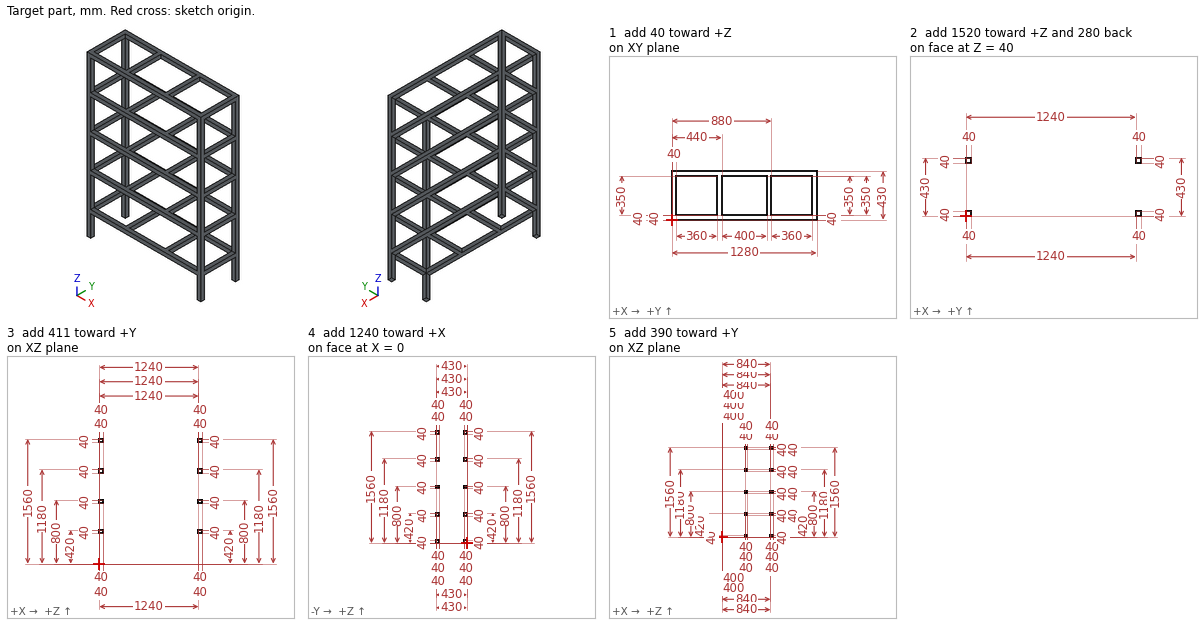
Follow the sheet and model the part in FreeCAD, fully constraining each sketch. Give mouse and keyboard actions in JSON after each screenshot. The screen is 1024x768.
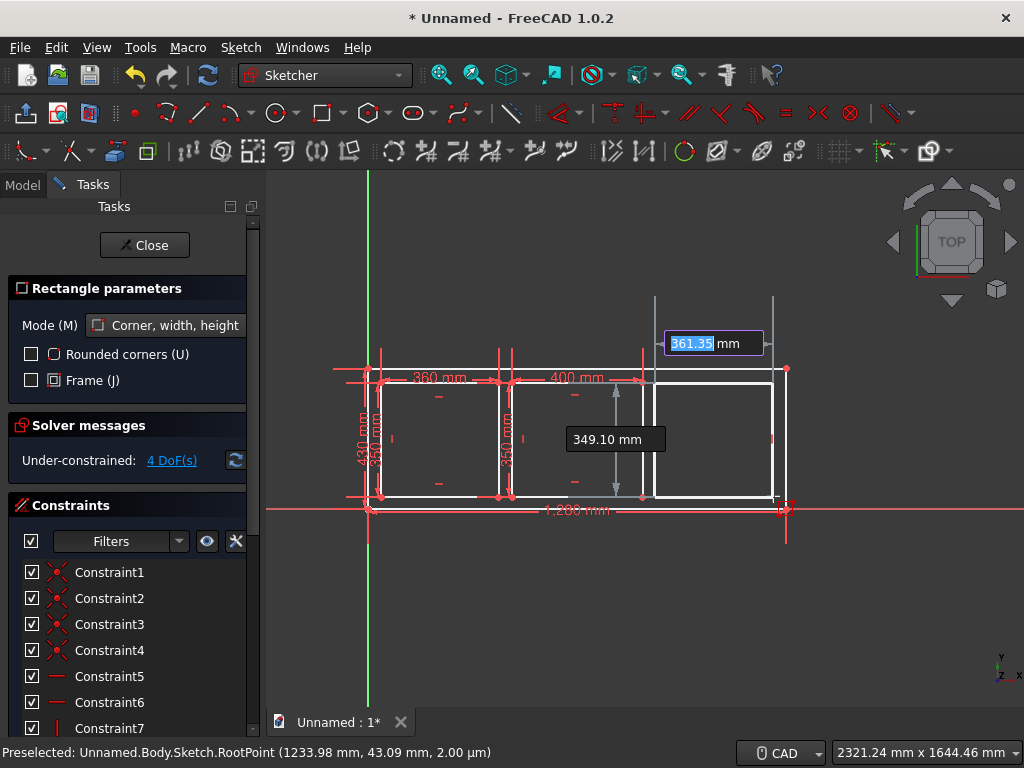
{"action": "type", "text": "360"}
{"action": "key", "text": "Tab"}
{"action": "type", "text": "350"}
{"action": "key", "text": "Return"}
{"action": "key", "text": "Escape"}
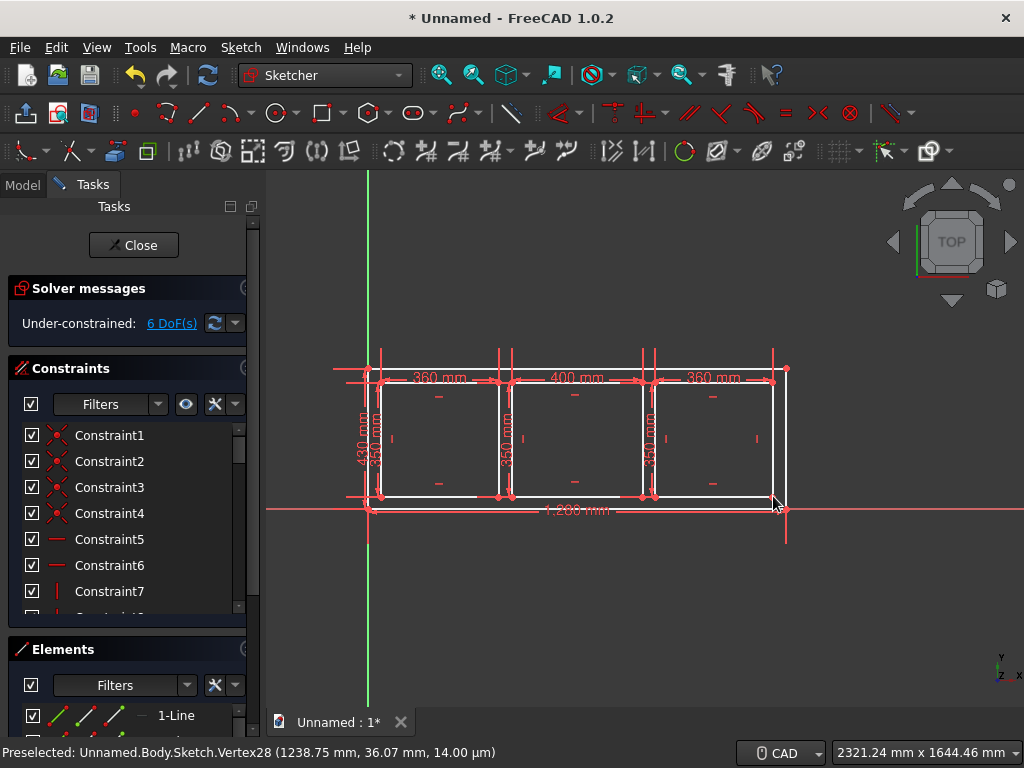
{"action": "left_click", "coordinate": [558, 114]}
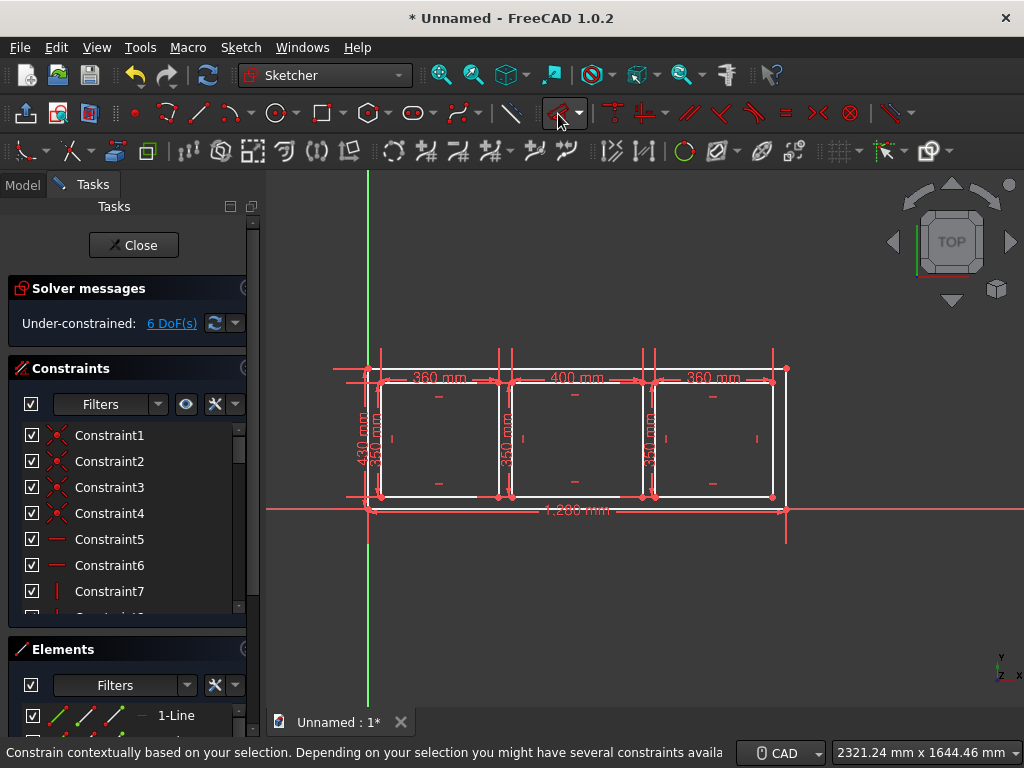
{"action": "scroll", "coordinate": [381, 383], "scroll_direction": "up", "scroll_amount": 6}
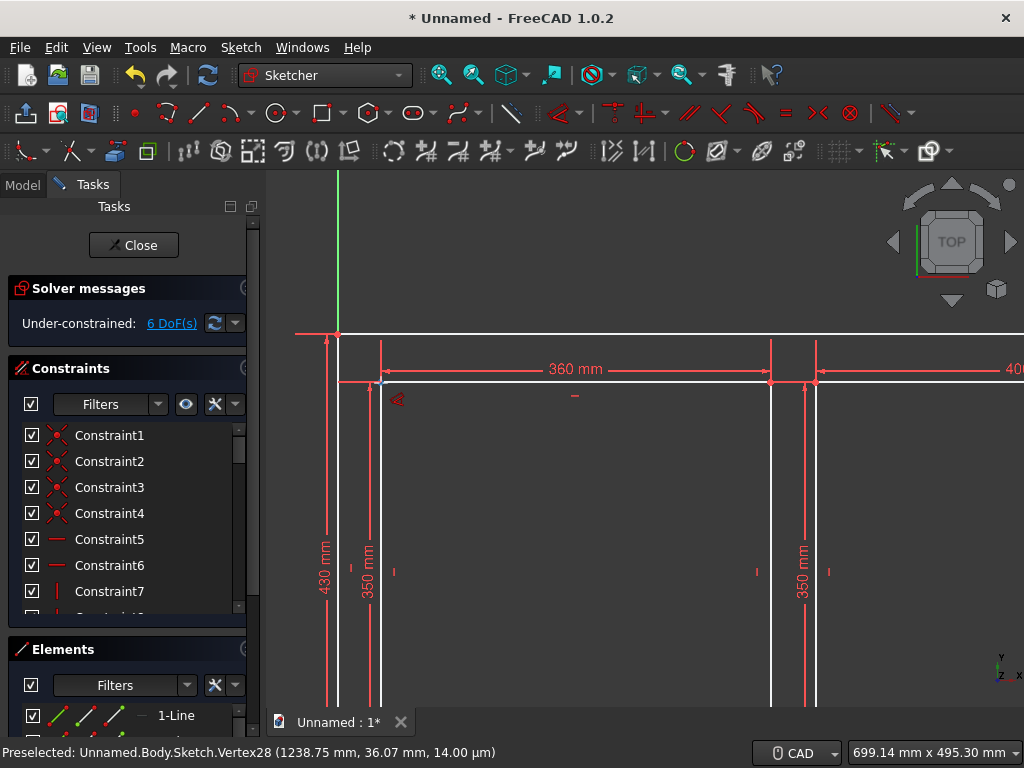
{"action": "left_click", "coordinate": [381, 382]}
{"action": "left_click", "coordinate": [359, 348]}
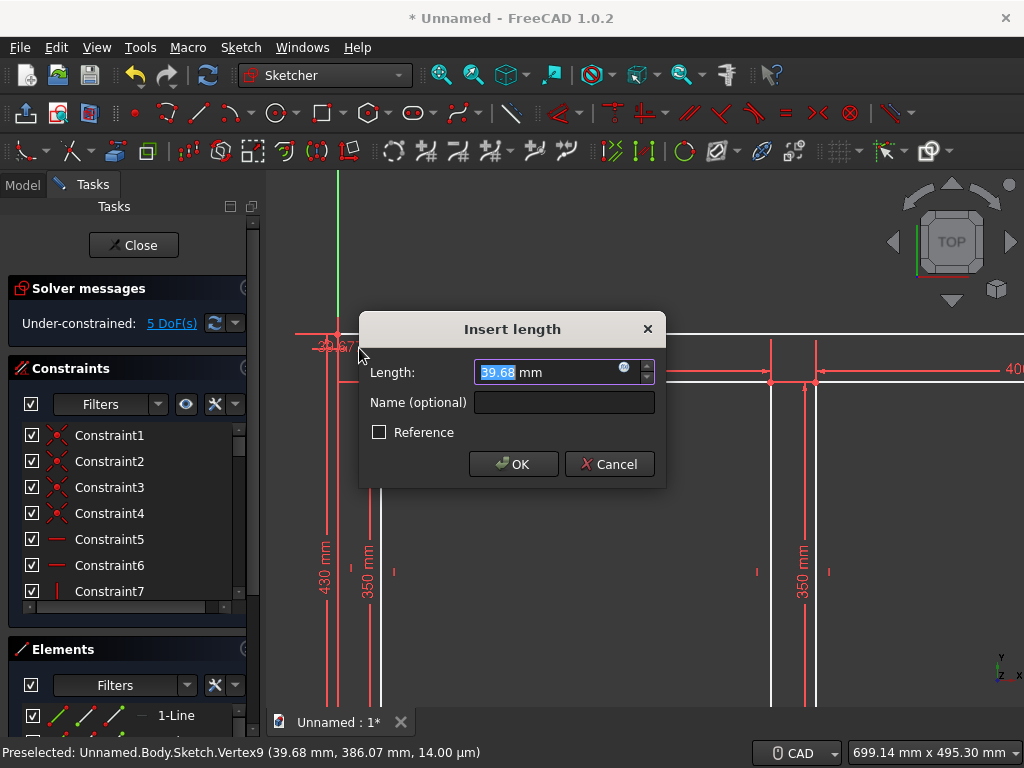
{"action": "type", "text": "40"}
{"action": "key", "text": "Return"}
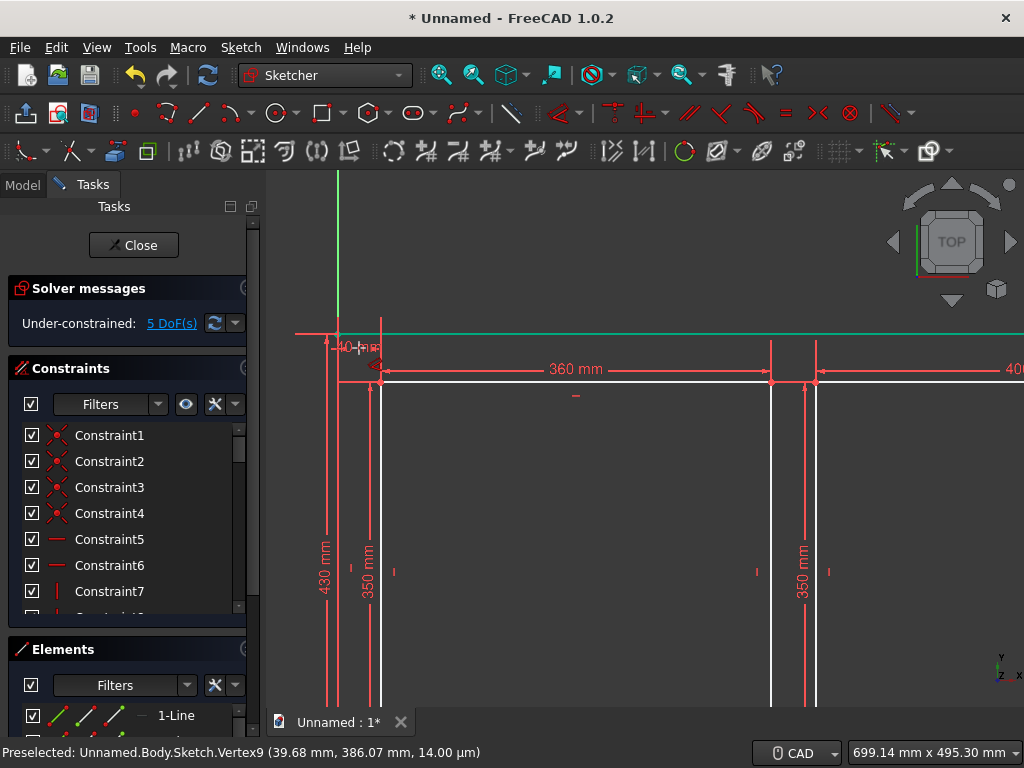
{"action": "scroll", "coordinate": [380, 383], "scroll_direction": "down", "scroll_amount": 6}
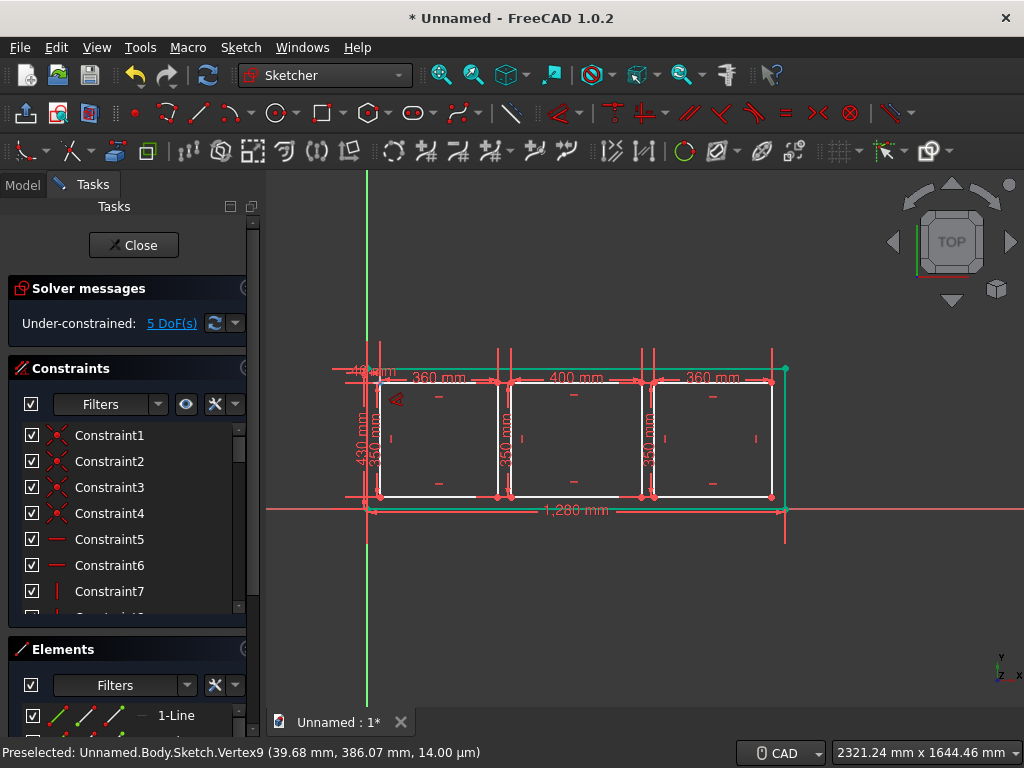
{"action": "scroll", "coordinate": [380, 497], "scroll_direction": "up", "scroll_amount": 6}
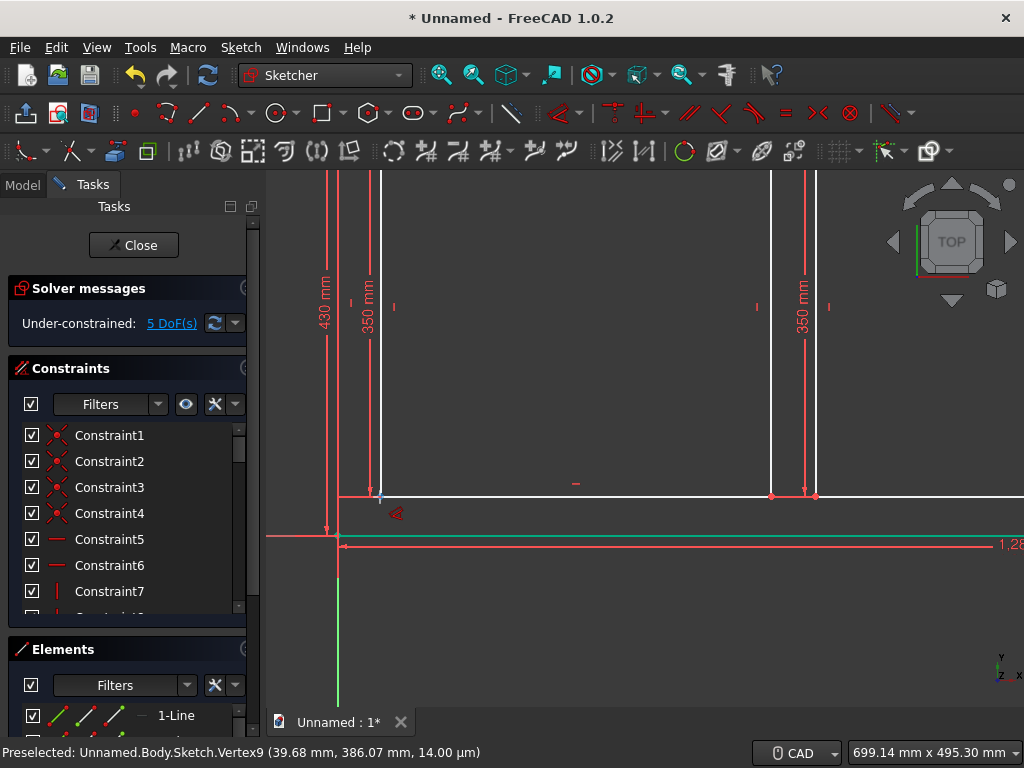
{"action": "left_click", "coordinate": [381, 497]}
{"action": "left_click", "coordinate": [304, 516]}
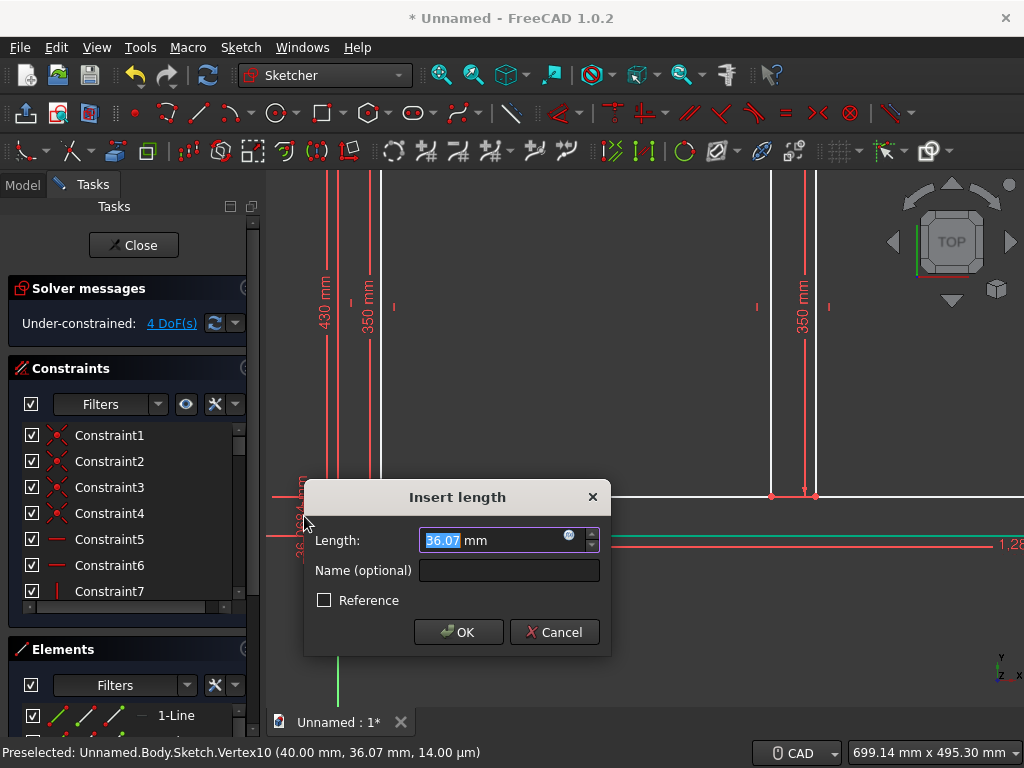
{"action": "type", "text": "40"}
{"action": "key", "text": "Return"}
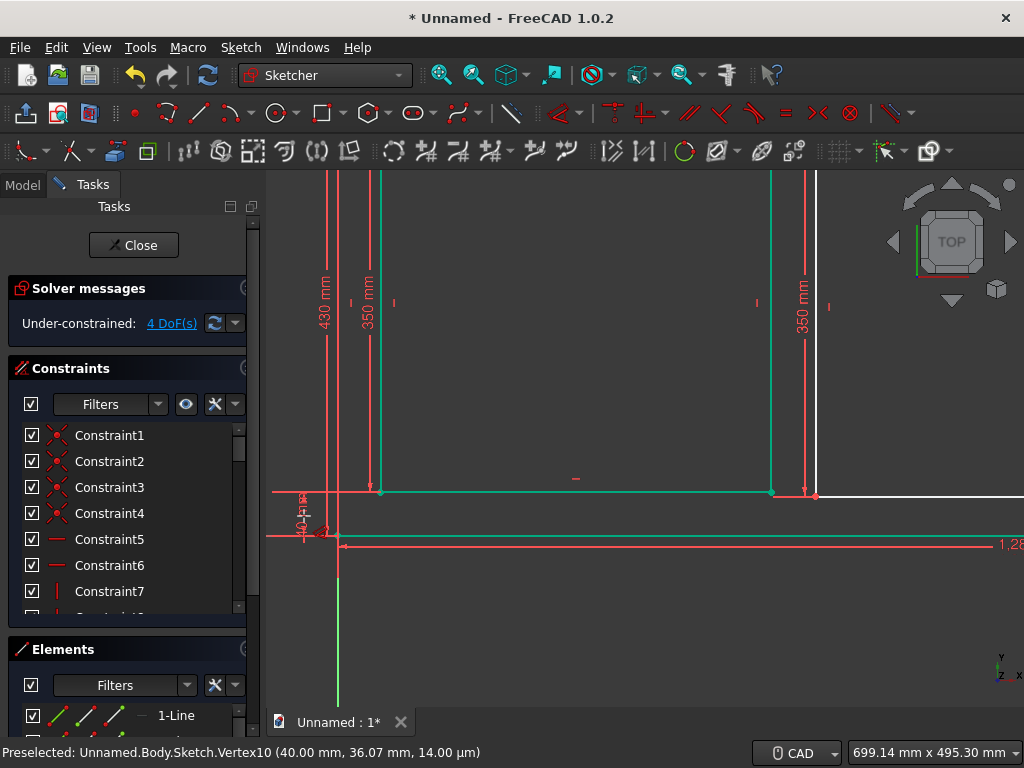
{"action": "left_click", "coordinate": [816, 497]}
{"action": "left_click", "coordinate": [850, 516]}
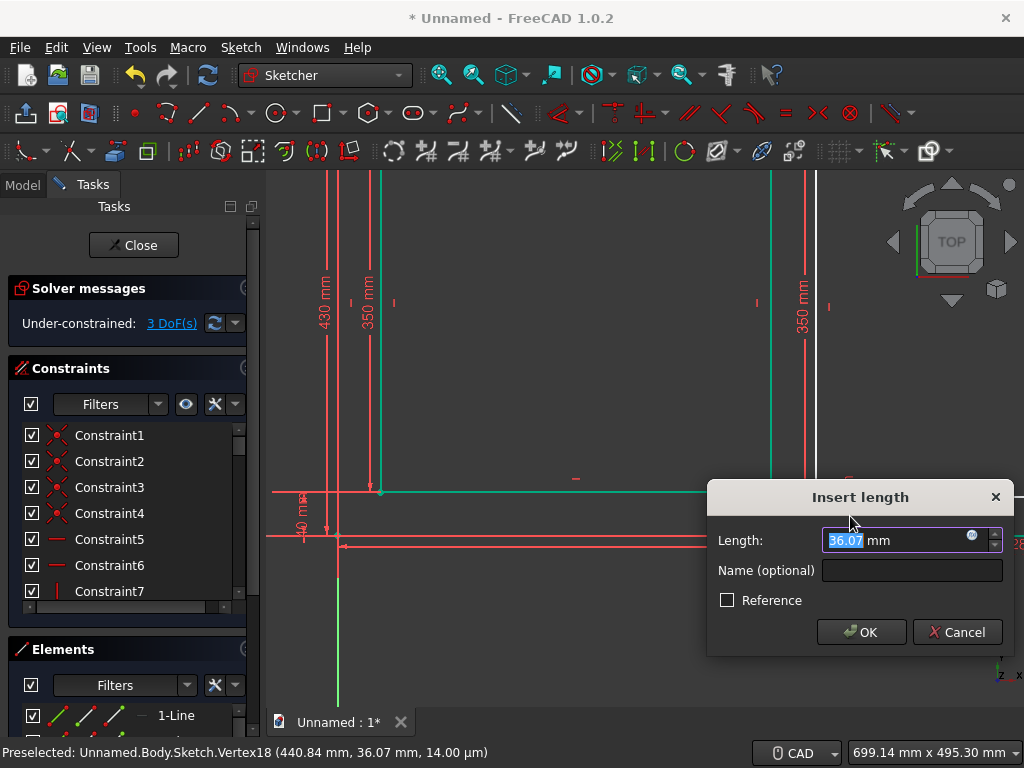
{"action": "type", "text": "40"}
{"action": "key", "text": "Return"}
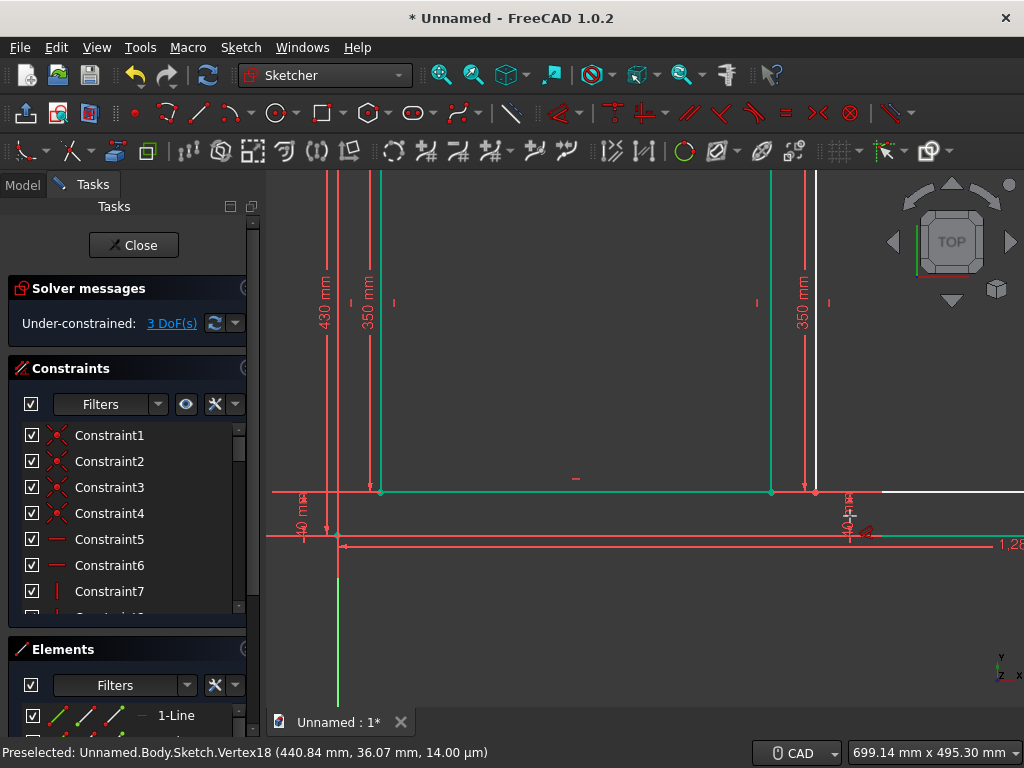
{"action": "scroll", "coordinate": [380, 497], "scroll_direction": "down", "scroll_amount": 6}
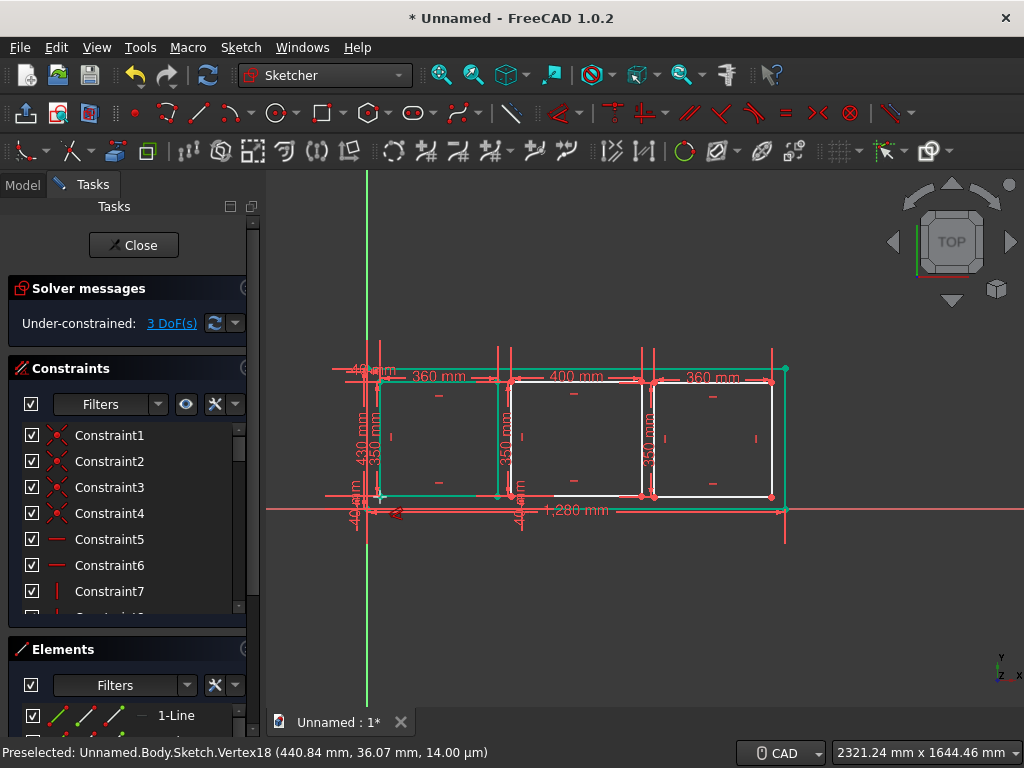
{"action": "scroll", "coordinate": [654, 497], "scroll_direction": "up", "scroll_amount": 6}